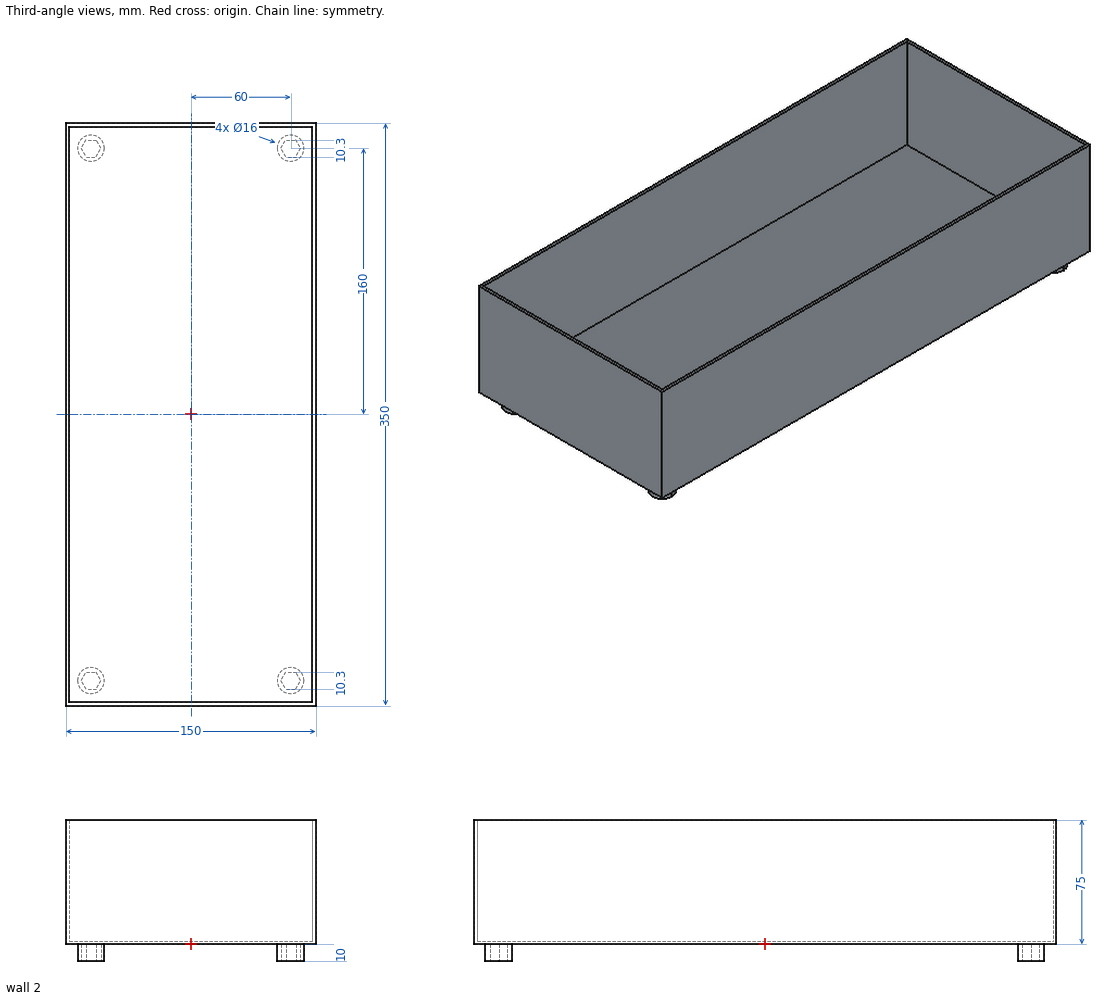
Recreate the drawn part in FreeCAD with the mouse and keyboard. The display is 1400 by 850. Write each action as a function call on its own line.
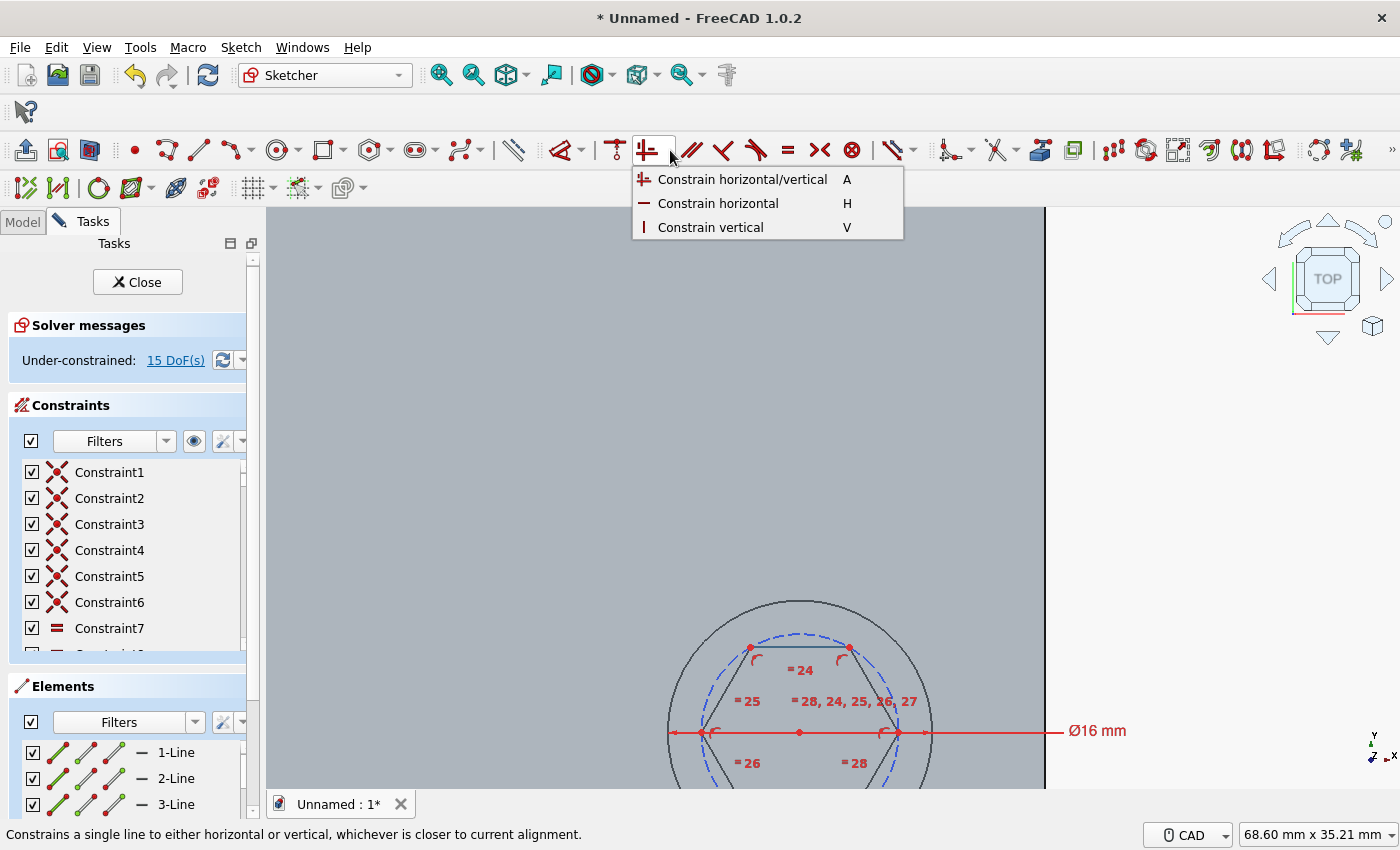
click(768, 203)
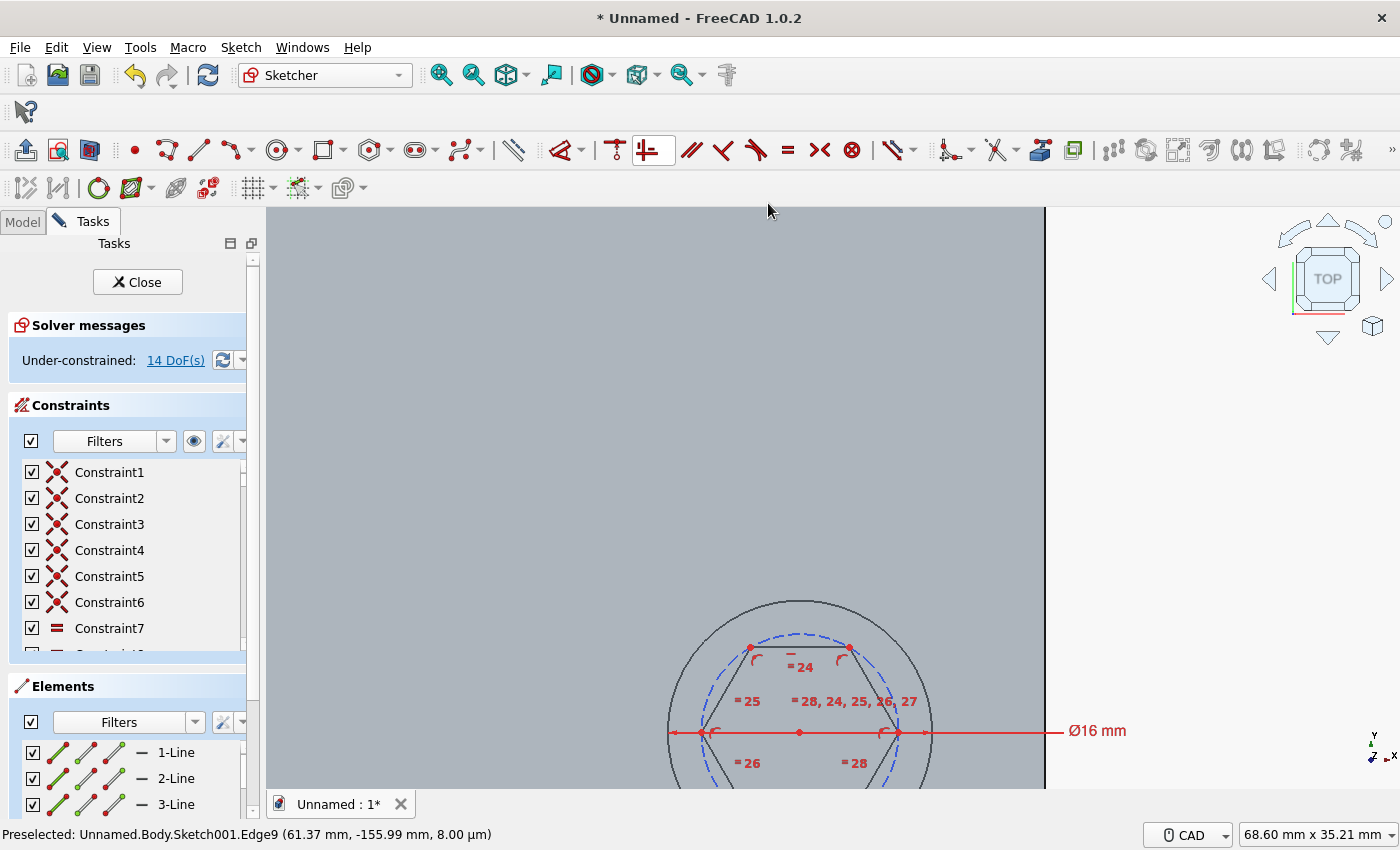
scroll(827, 655, down, 14)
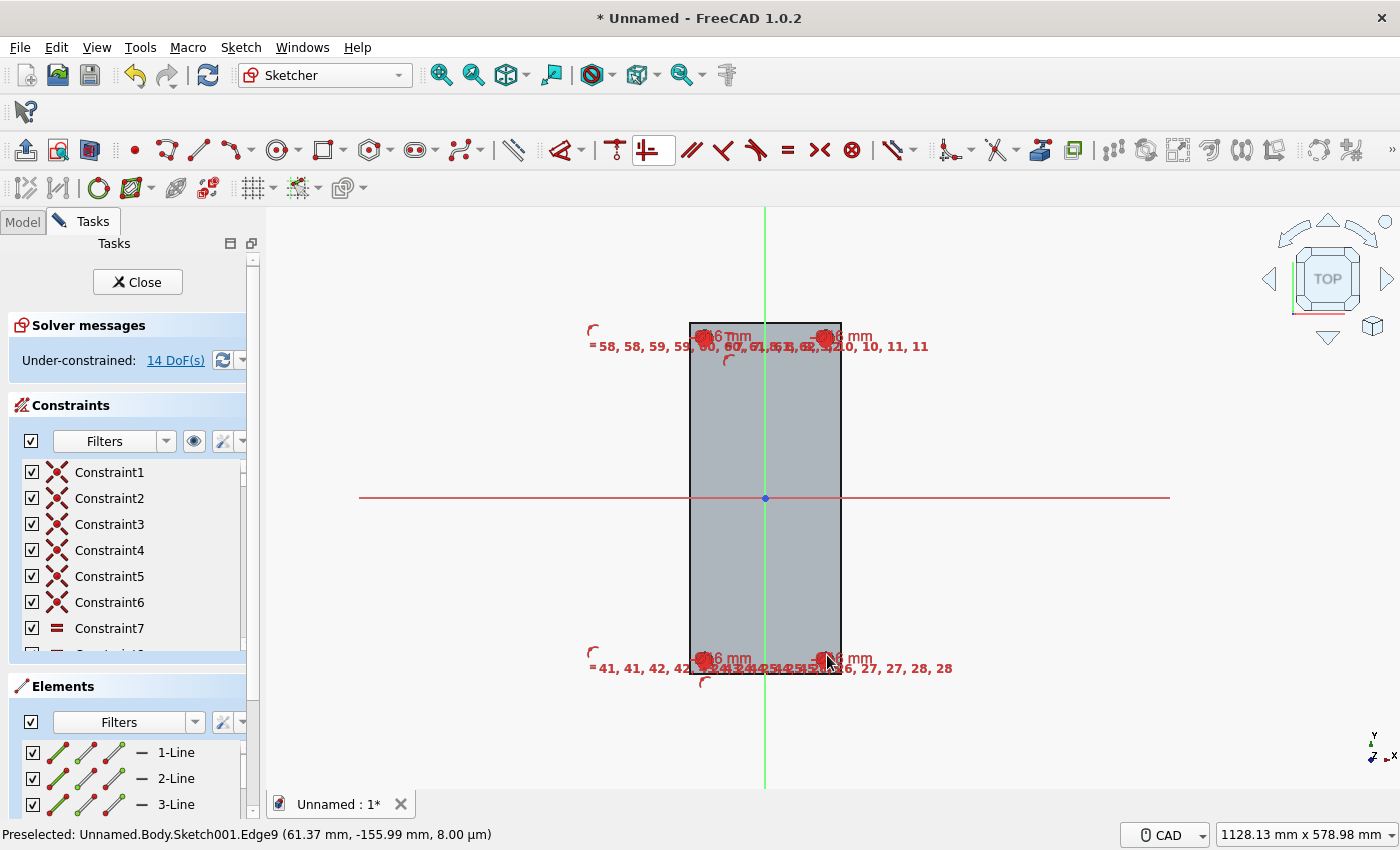
scroll(704, 666, up, 14)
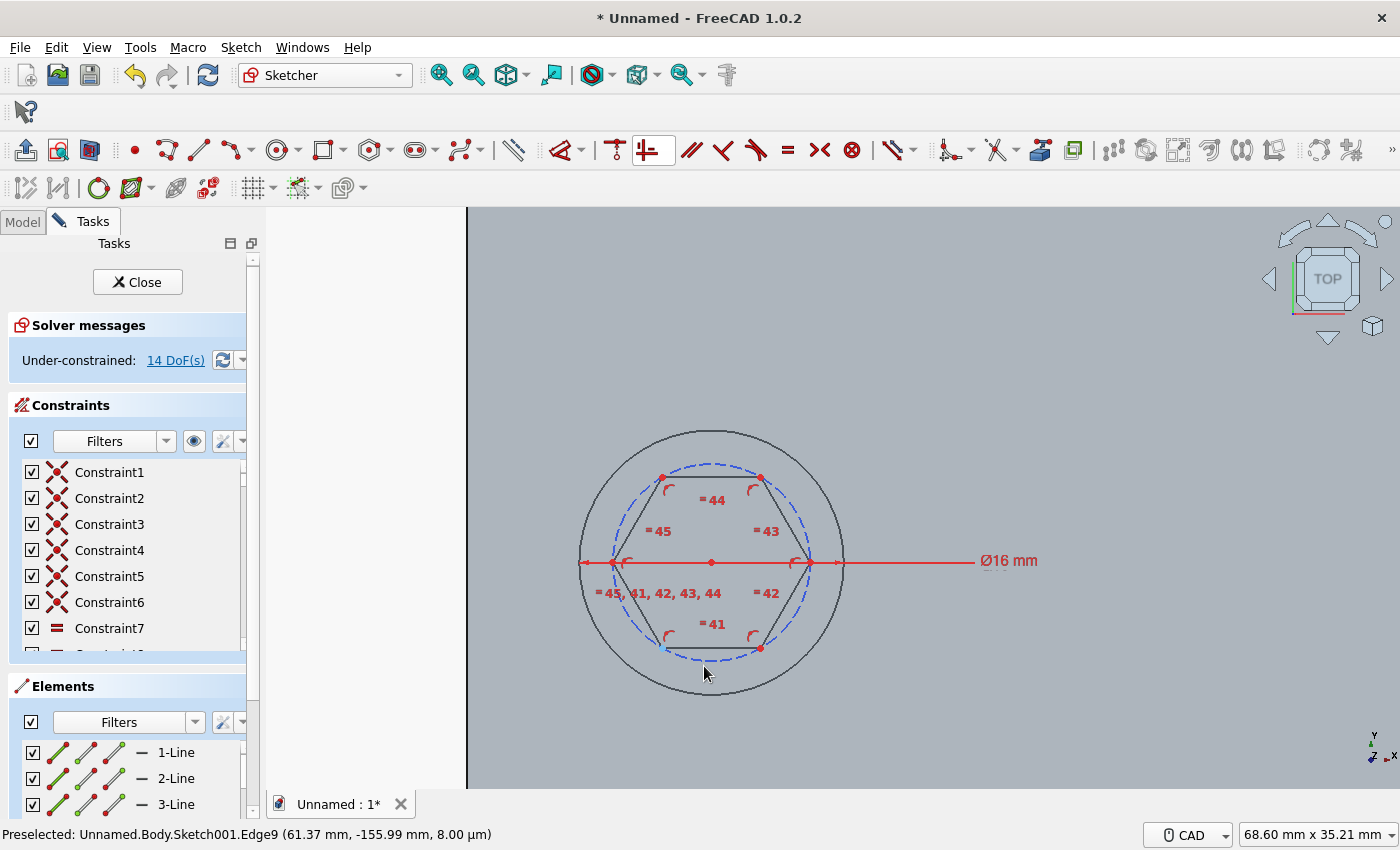
click(692, 648)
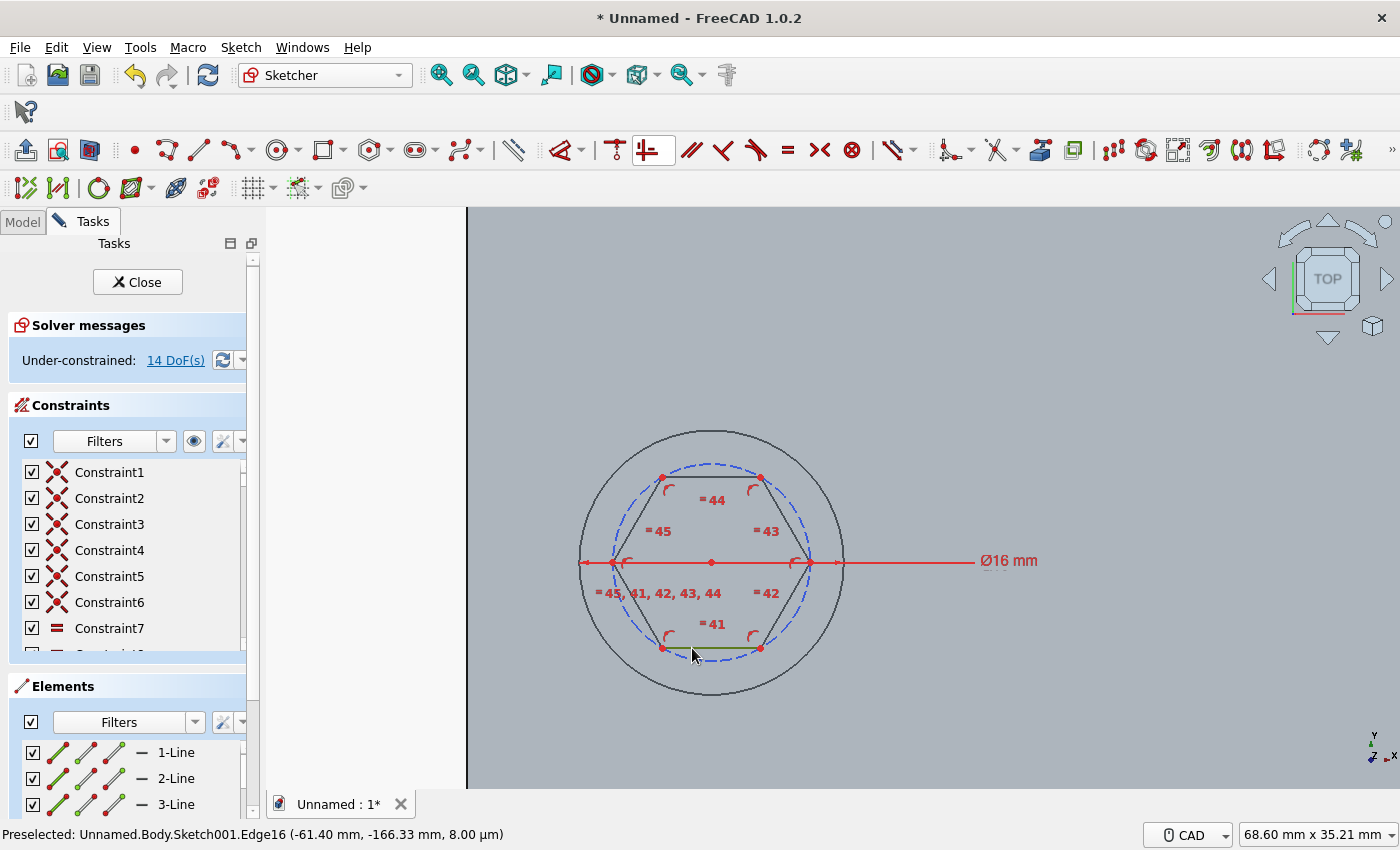
click(670, 150)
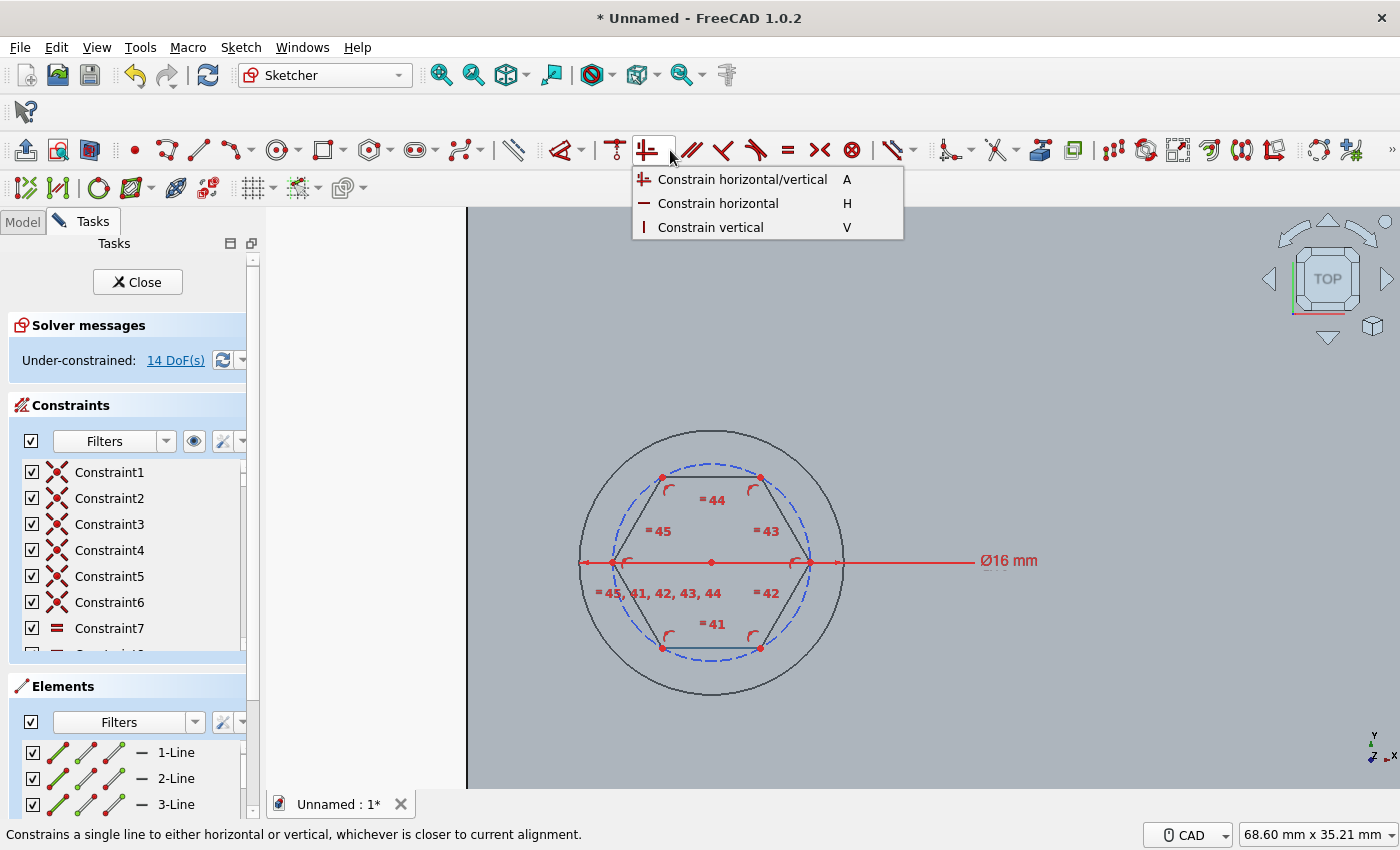
click(768, 203)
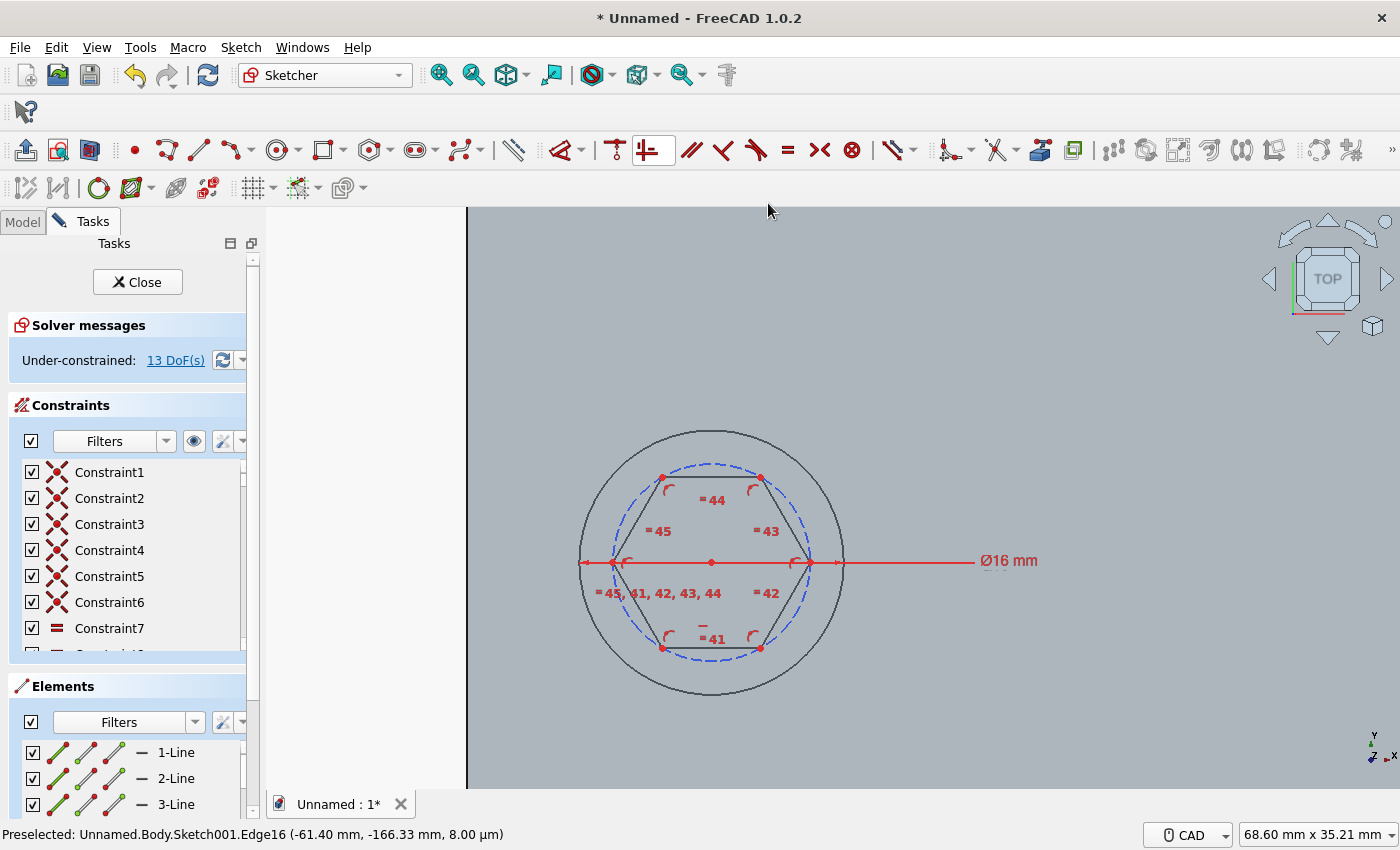
scroll(703, 666, down, 14)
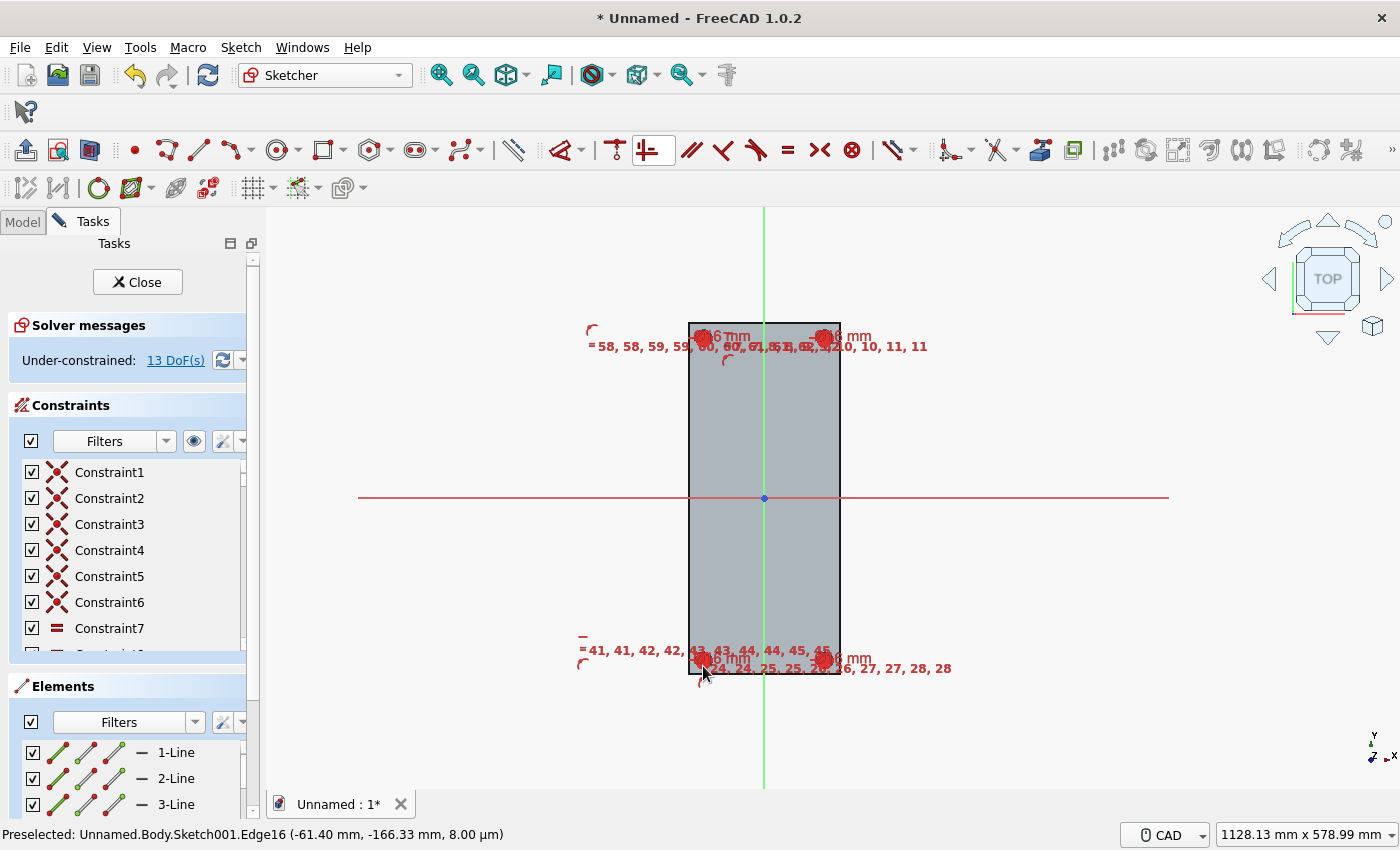
scroll(703, 343, up, 14)